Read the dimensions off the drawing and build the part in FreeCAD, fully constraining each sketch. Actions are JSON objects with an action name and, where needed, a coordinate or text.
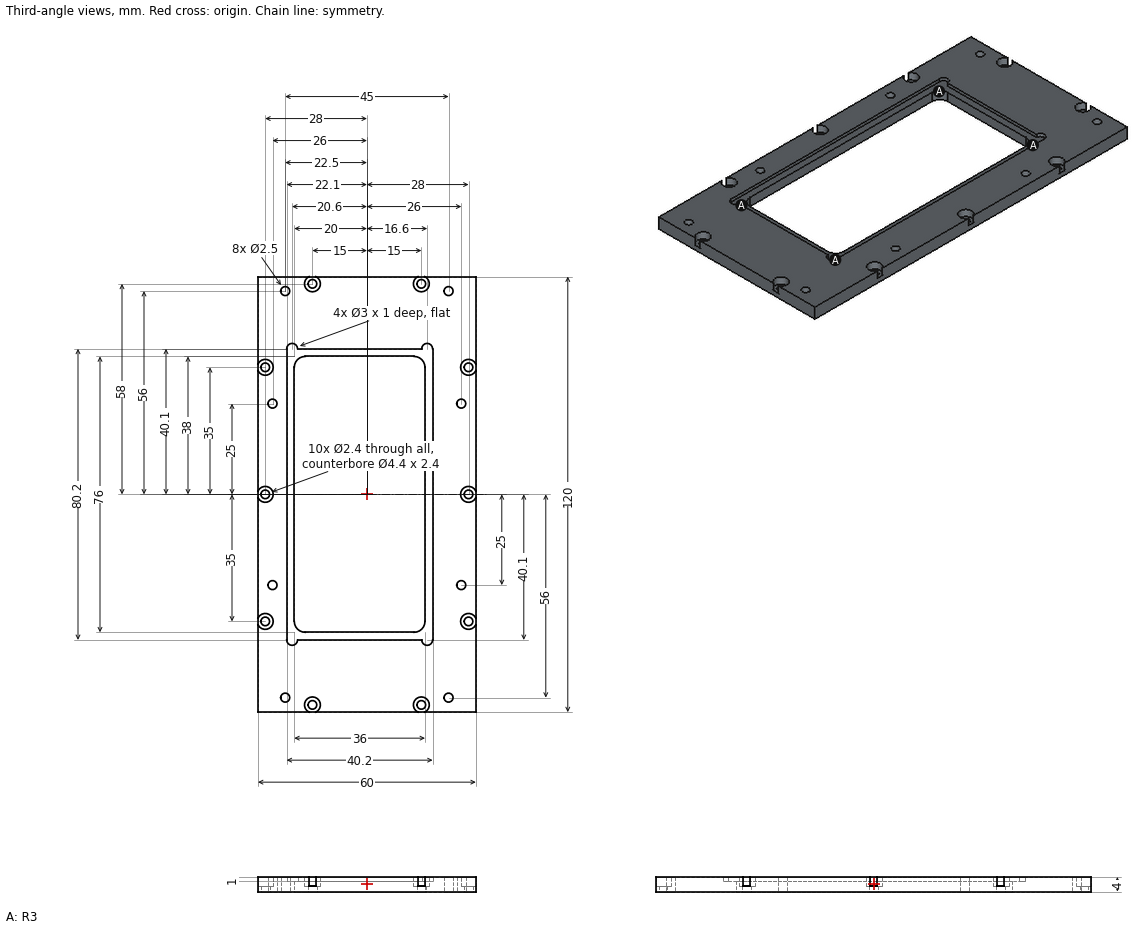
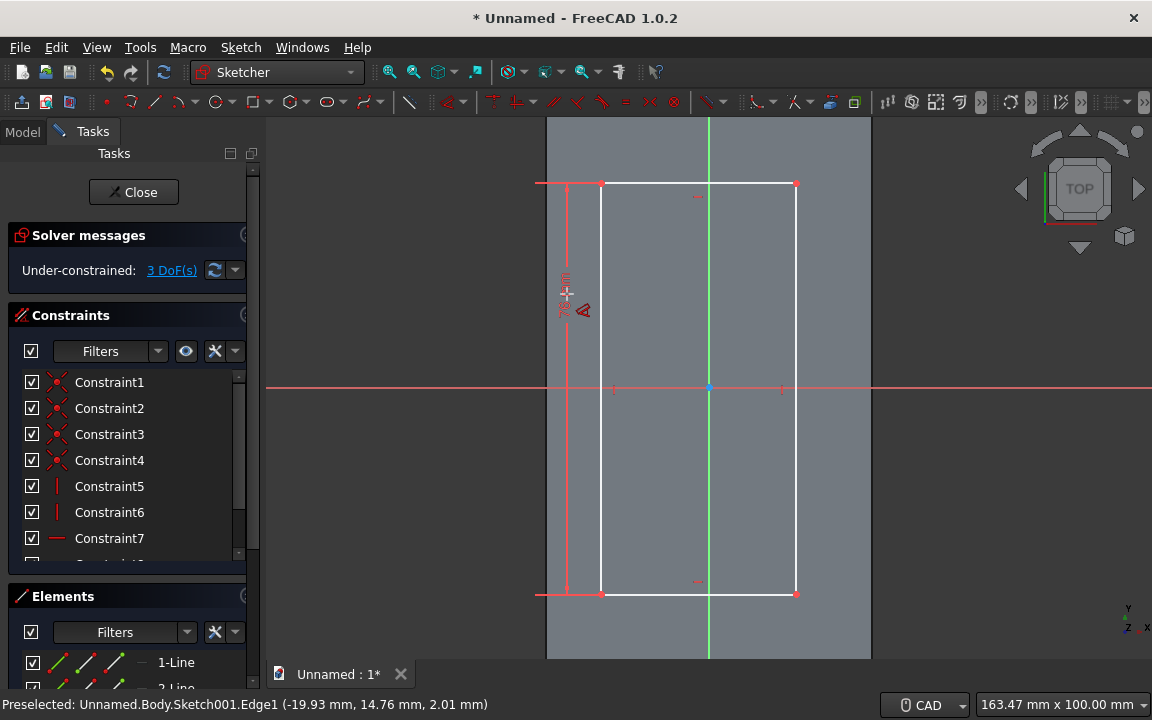
{"action": "left_click", "coordinate": [660, 595]}
{"action": "left_click", "coordinate": [654, 629]}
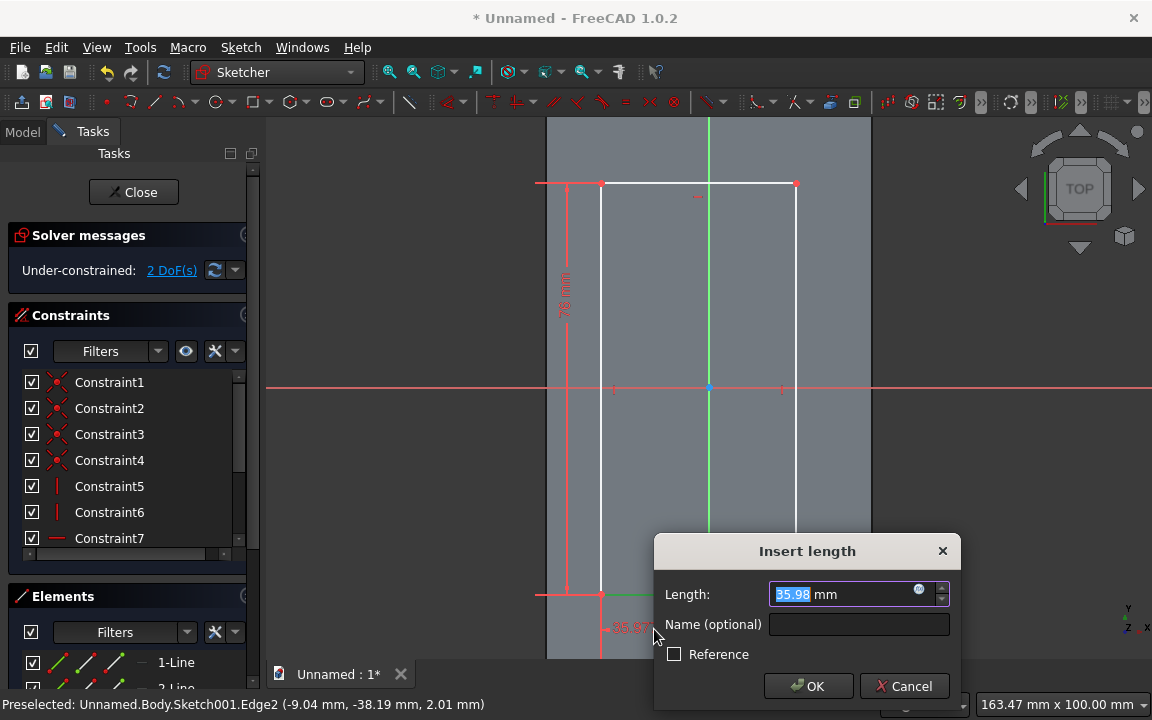
{"action": "type", "text": "36"}
{"action": "key", "text": "Return"}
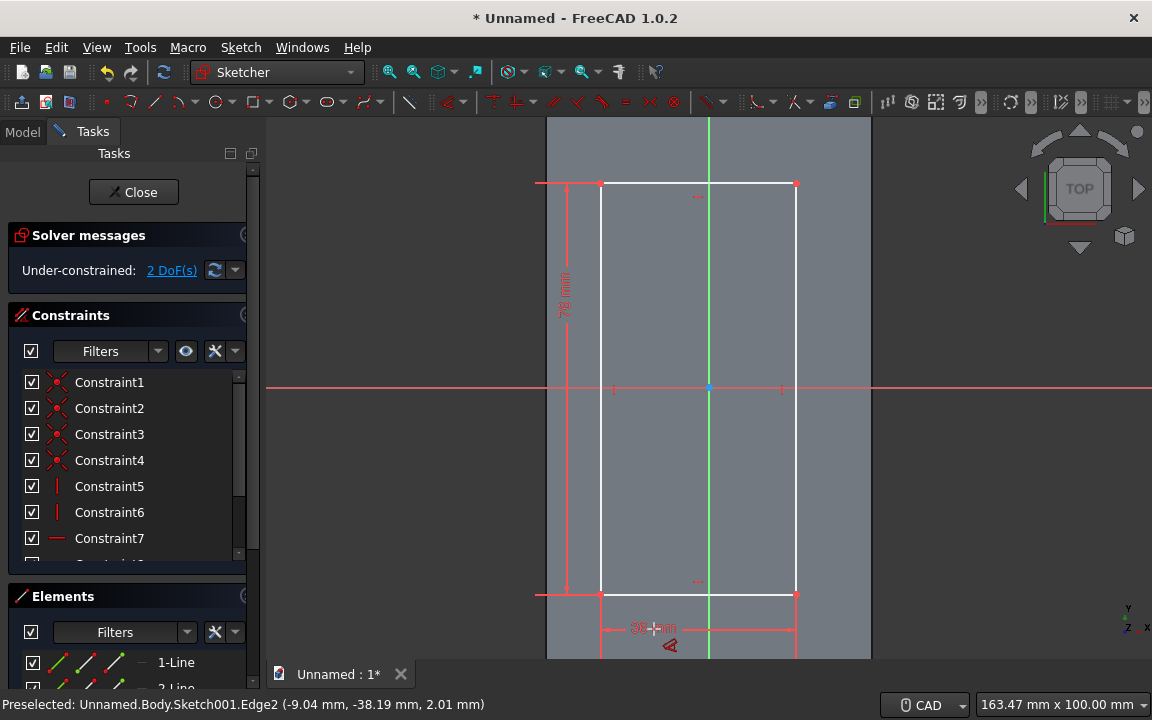
{"action": "left_click", "coordinate": [601, 183]}
{"action": "left_click", "coordinate": [655, 149]}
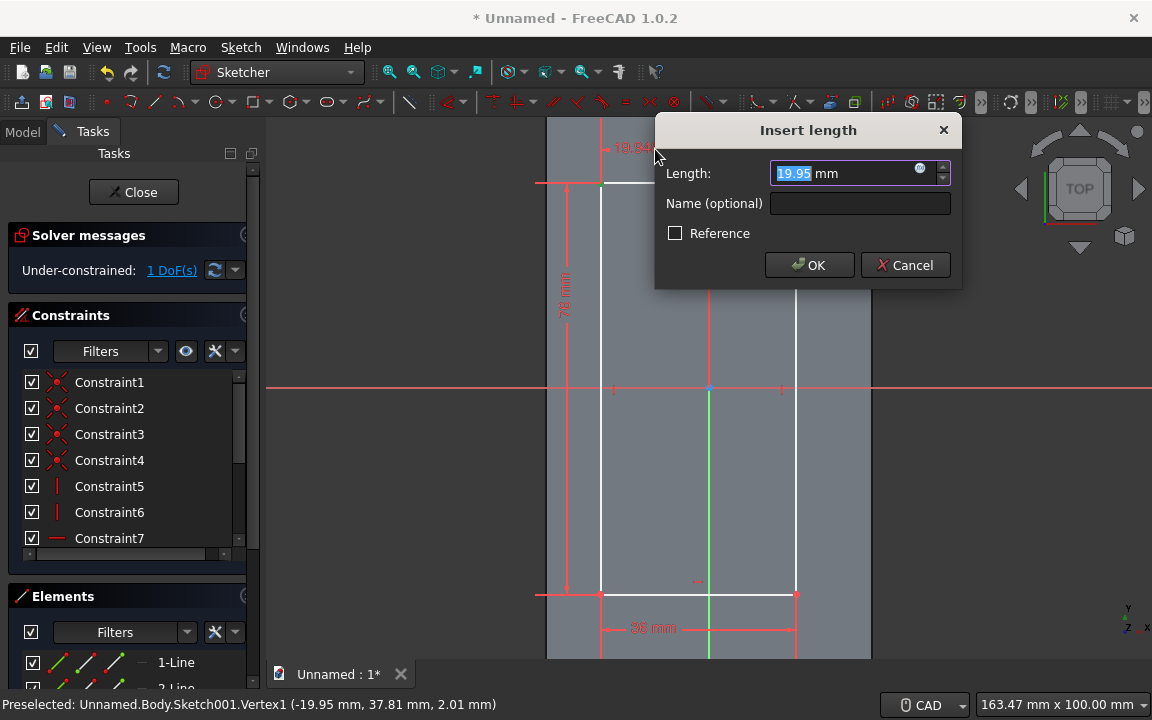
{"action": "type", "text": "20"}
{"action": "key", "text": "Return"}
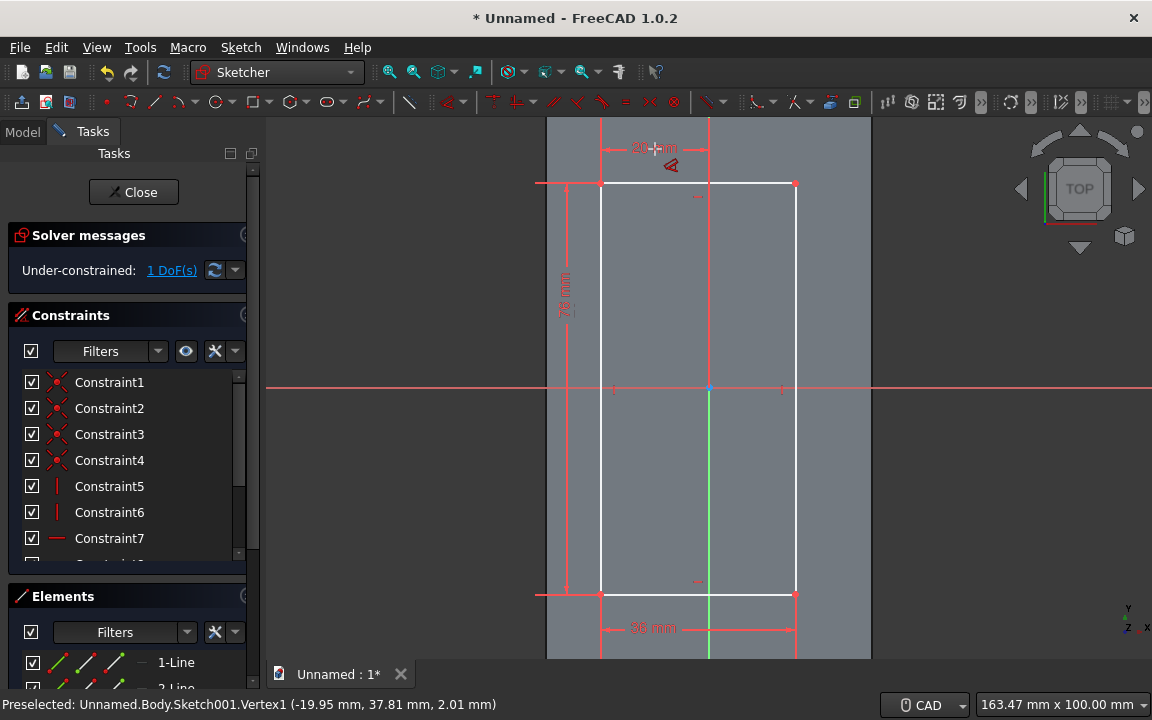
{"action": "left_click", "coordinate": [601, 183]}
{"action": "left_click", "coordinate": [567, 238]}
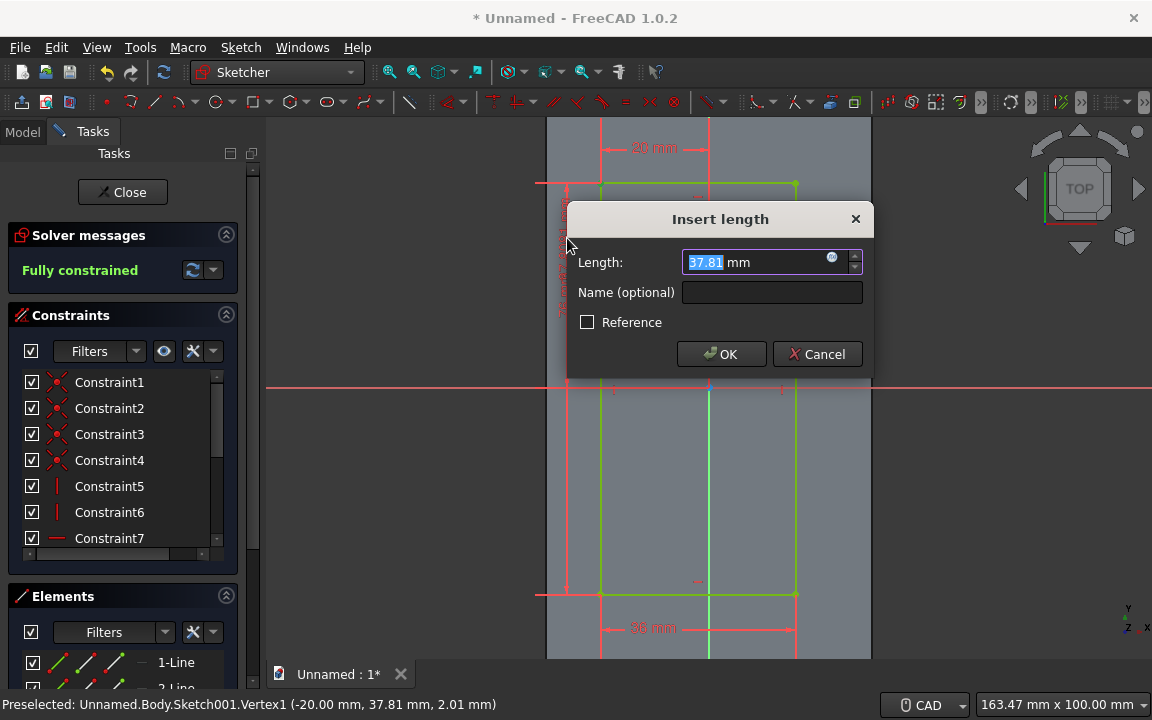
{"action": "type", "text": "38"}
{"action": "key", "text": "Return"}
{"action": "key", "text": "Escape"}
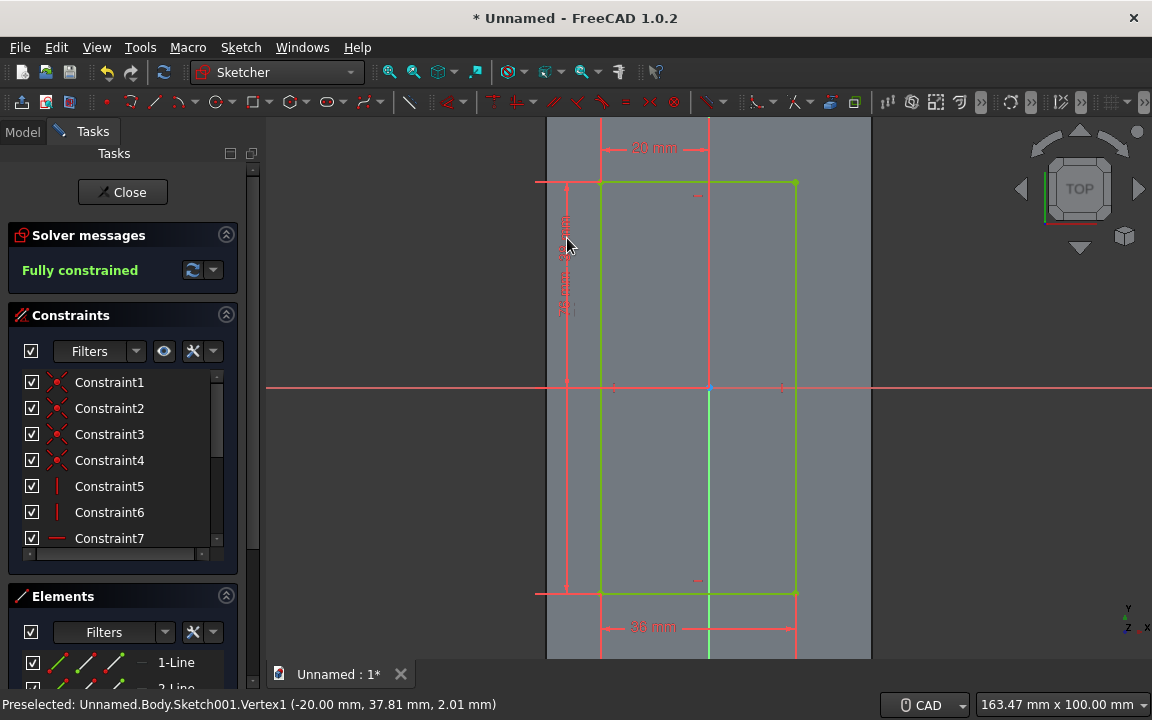
{"action": "left_click", "coordinate": [123, 192]}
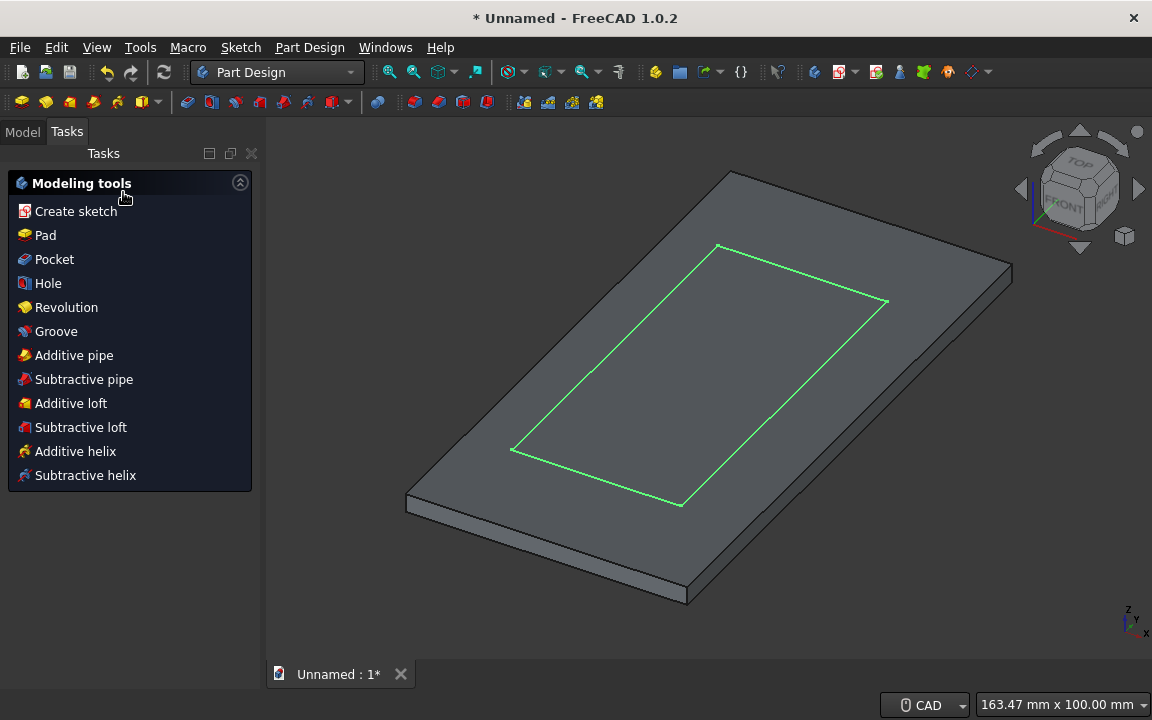
{"action": "left_click", "coordinate": [188, 102]}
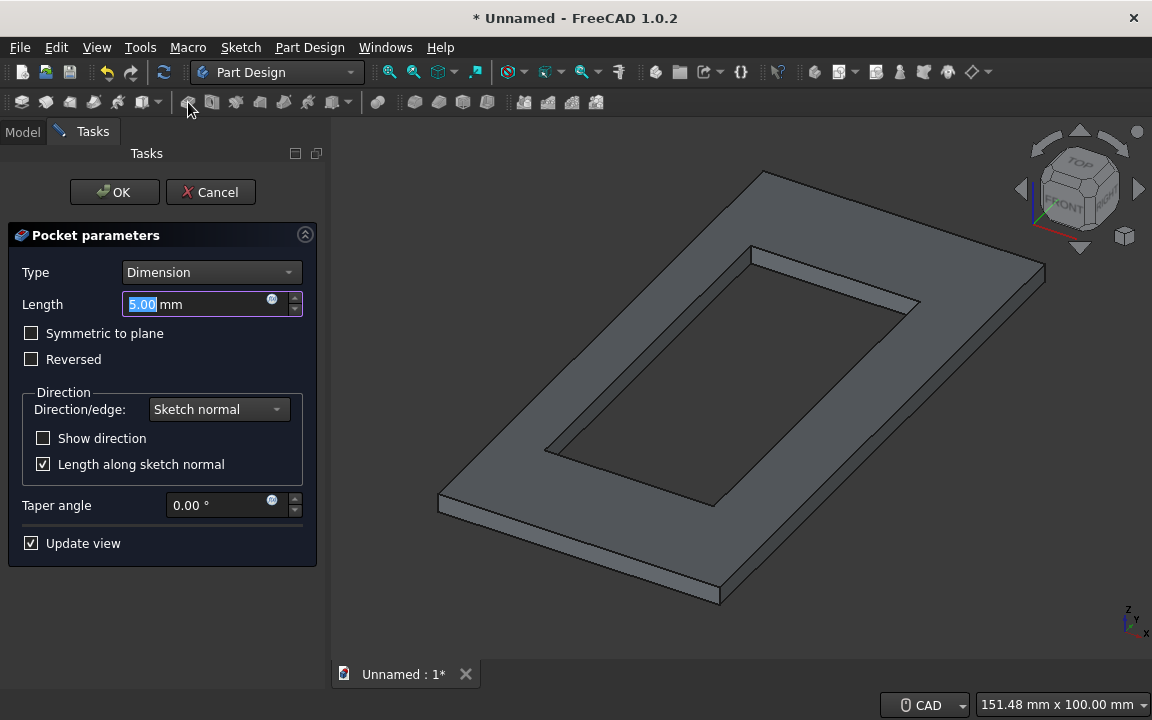
{"action": "left_click", "coordinate": [212, 272]}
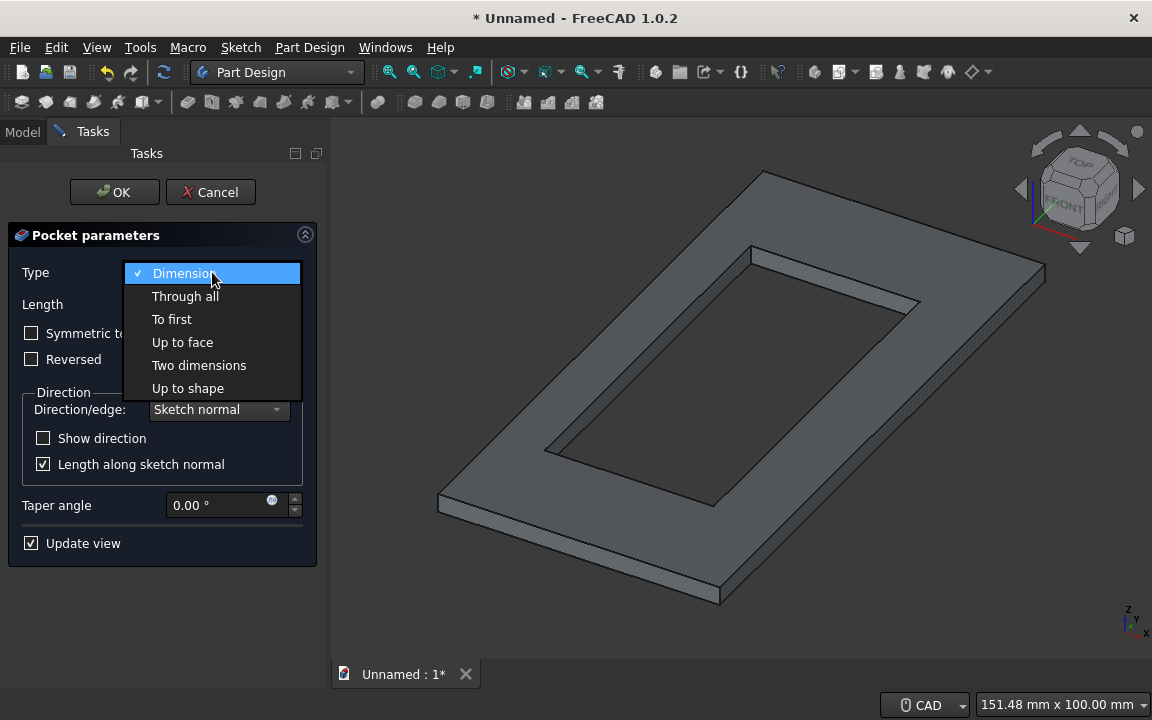
{"action": "left_click", "coordinate": [212, 296]}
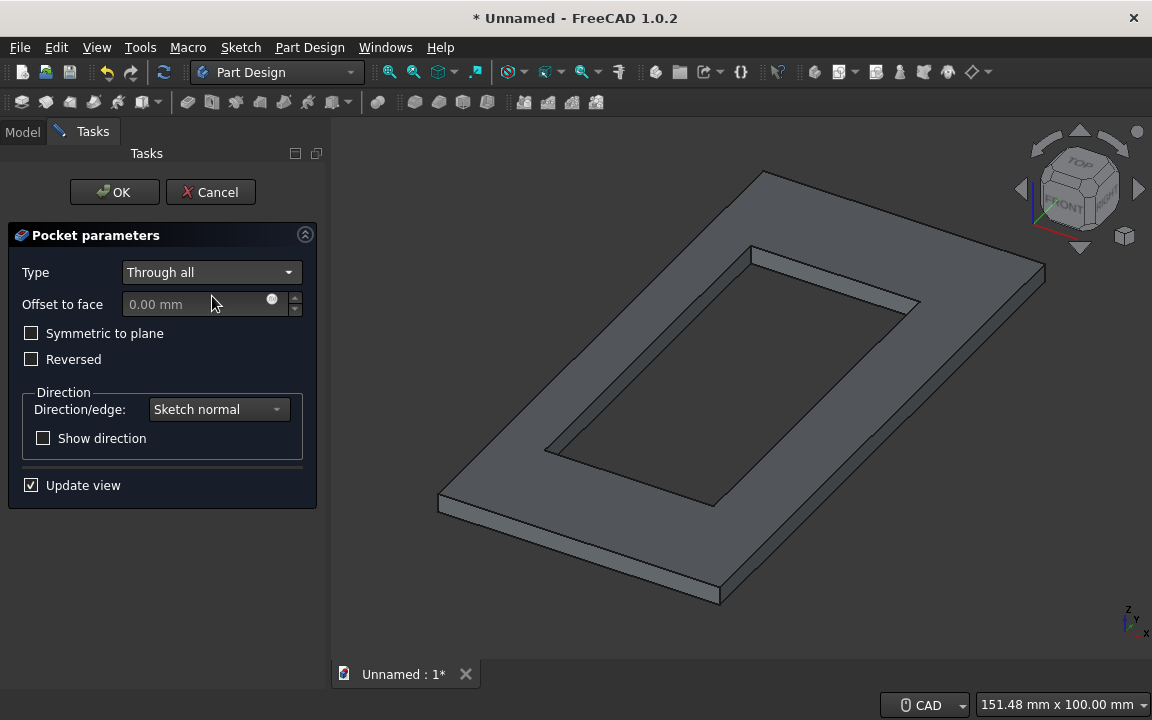
{"action": "left_click", "coordinate": [115, 192]}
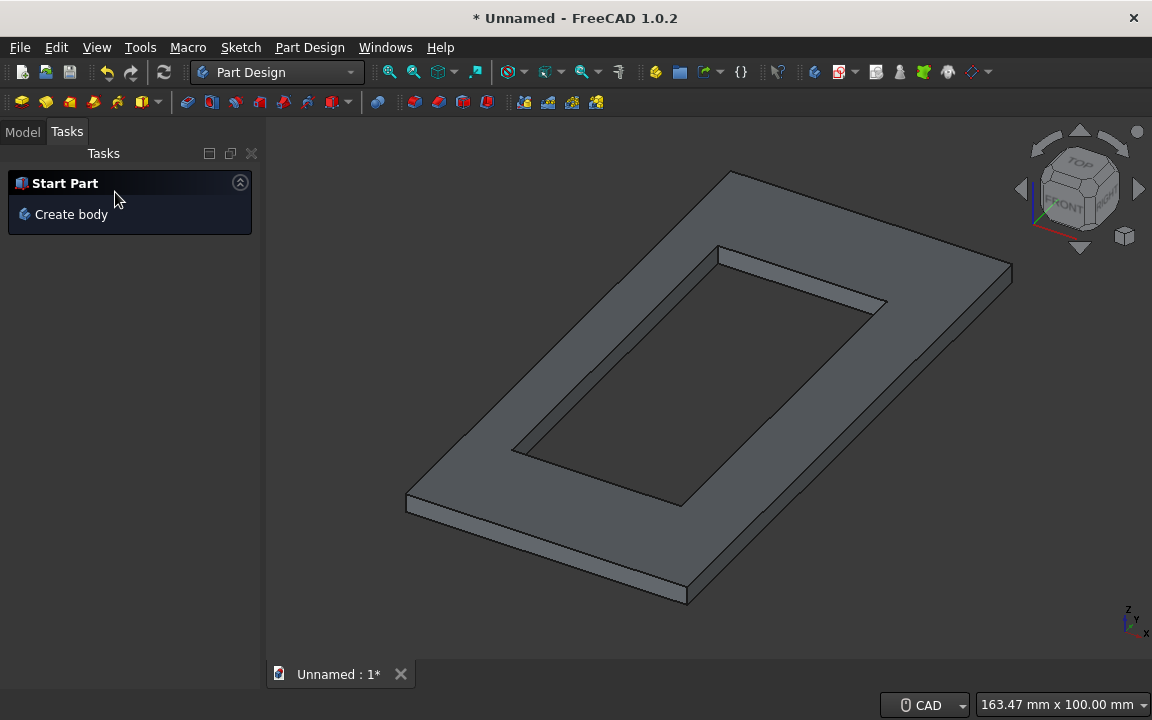
{"action": "left_click", "coordinate": [929, 266]}